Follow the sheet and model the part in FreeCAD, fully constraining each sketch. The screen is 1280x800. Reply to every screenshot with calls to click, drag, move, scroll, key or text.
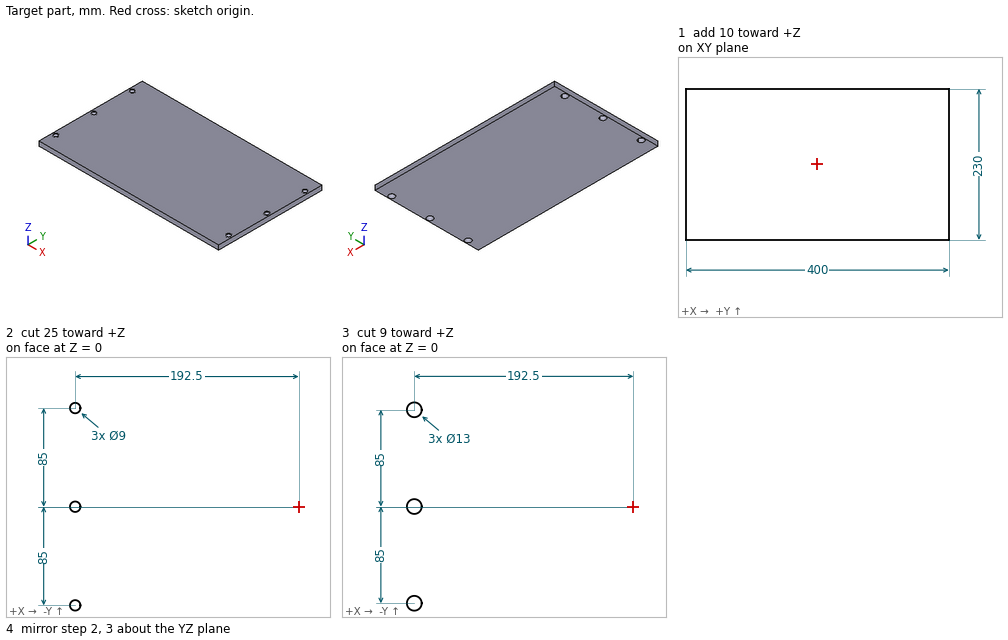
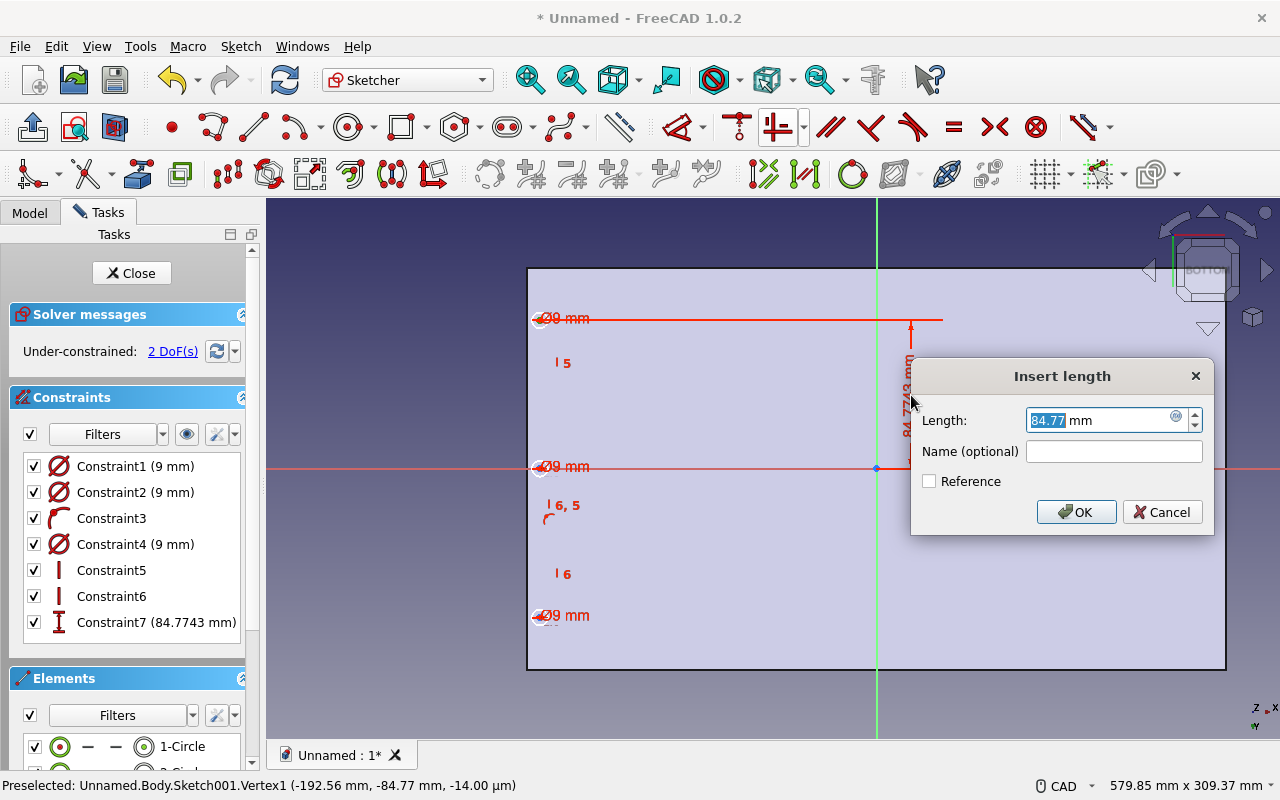
text(85)
key(Return)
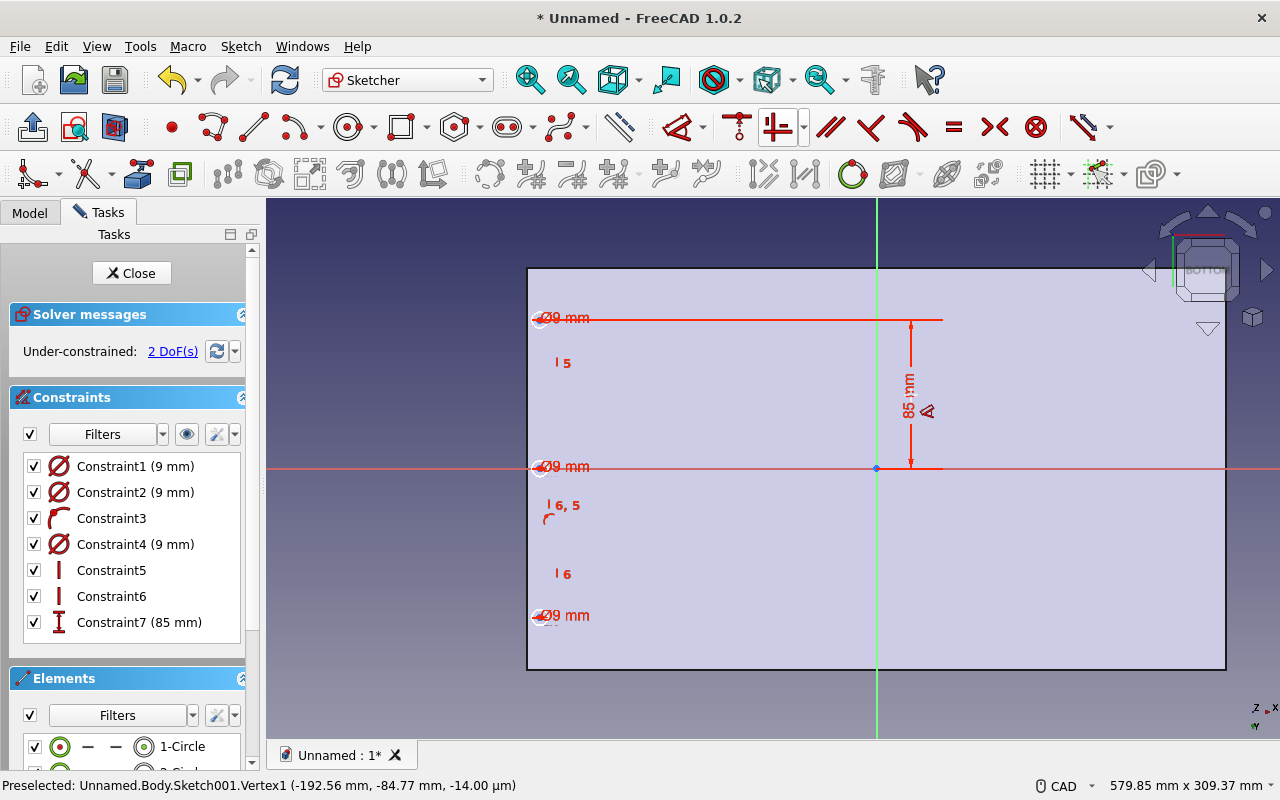
click(540, 618)
click(911, 543)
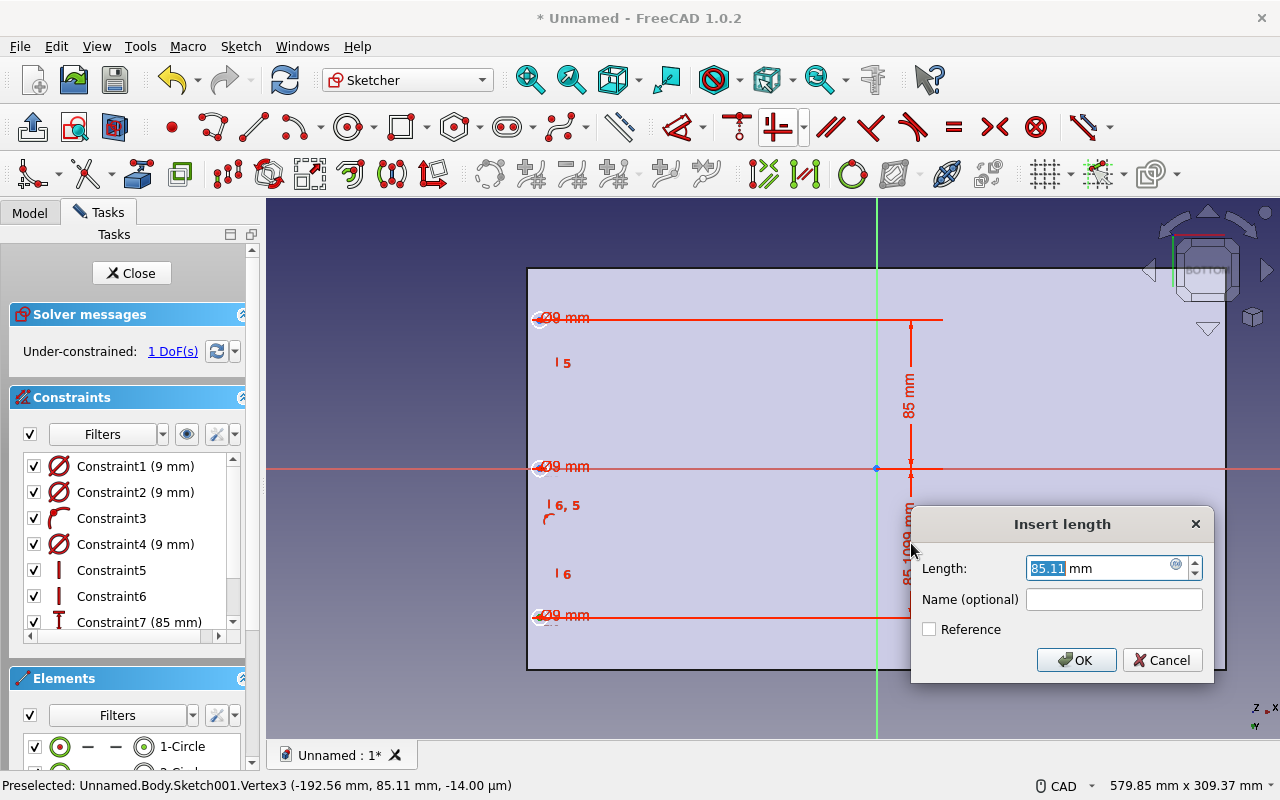
text(85)
key(Return)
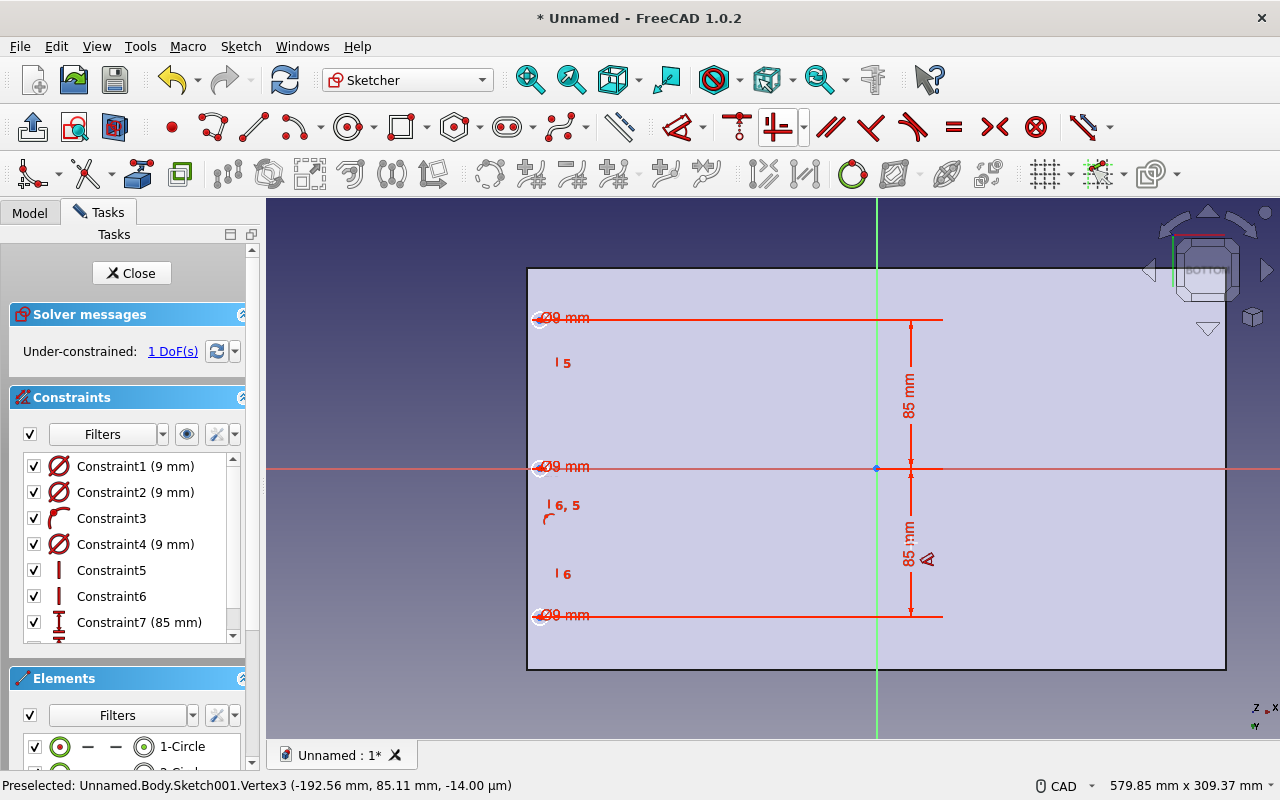
click(540, 320)
click(708, 286)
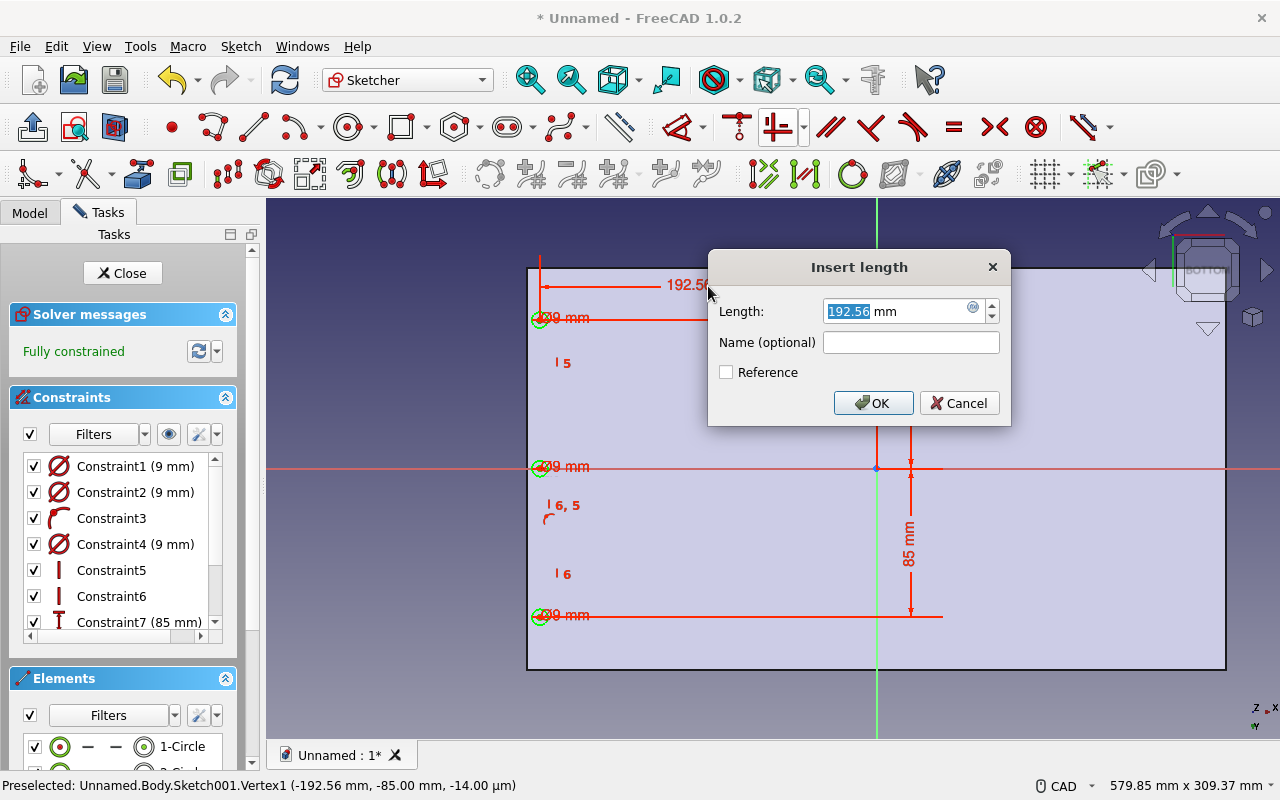
text(192.5)
key(Return)
key(Escape)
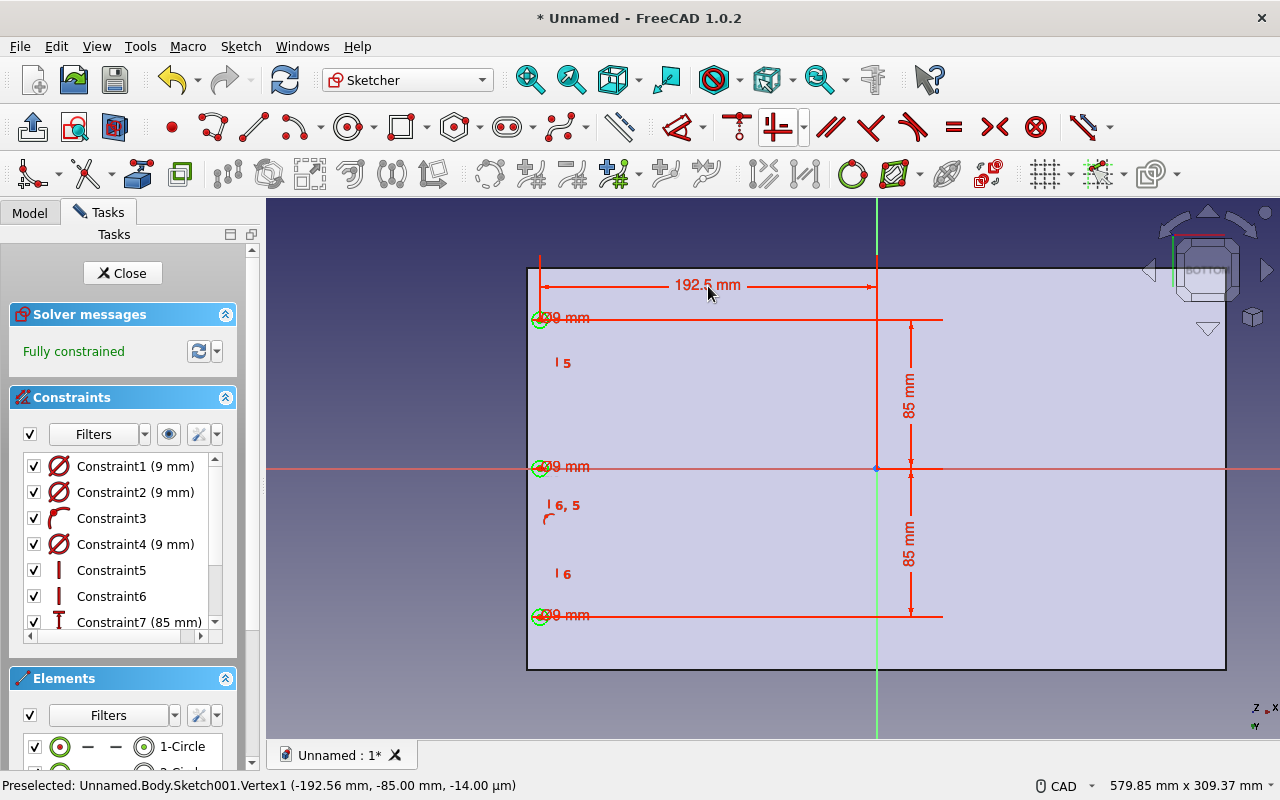
click(123, 273)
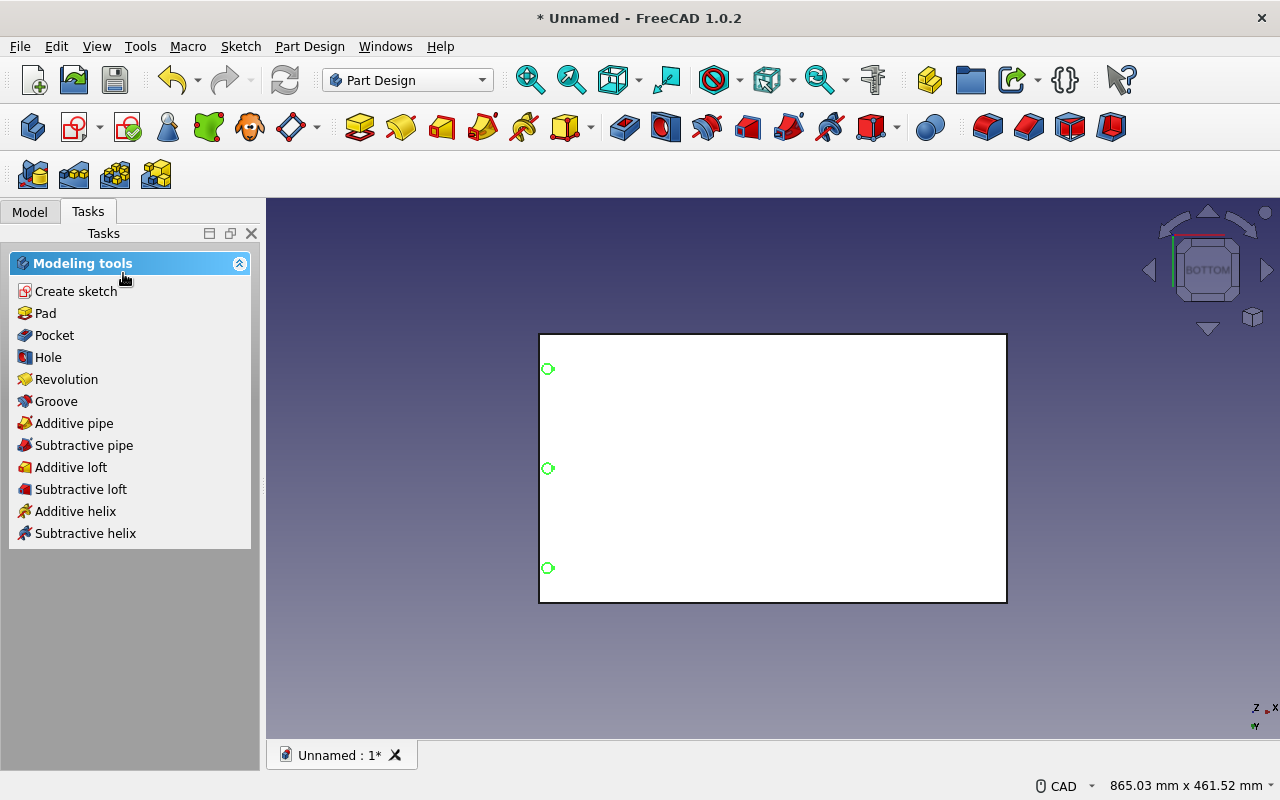
click(625, 128)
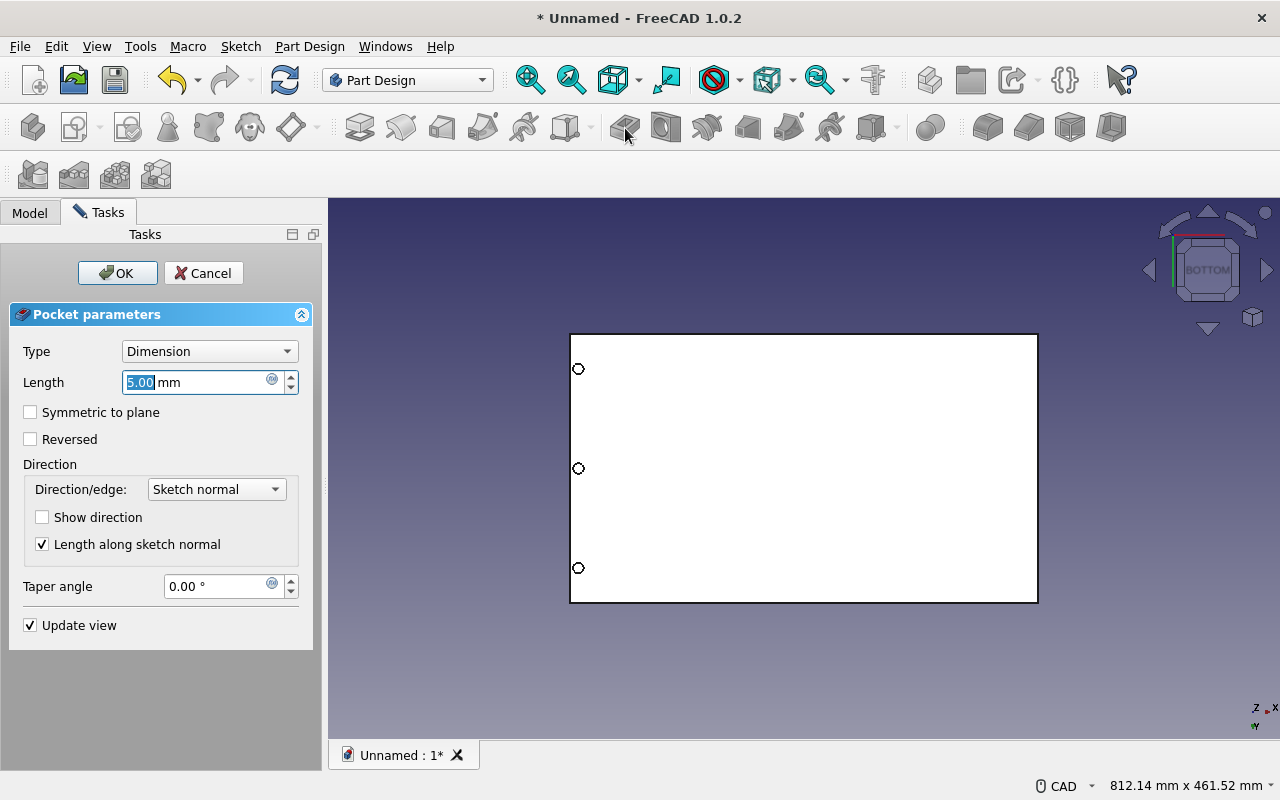
text(25)
key(Tab)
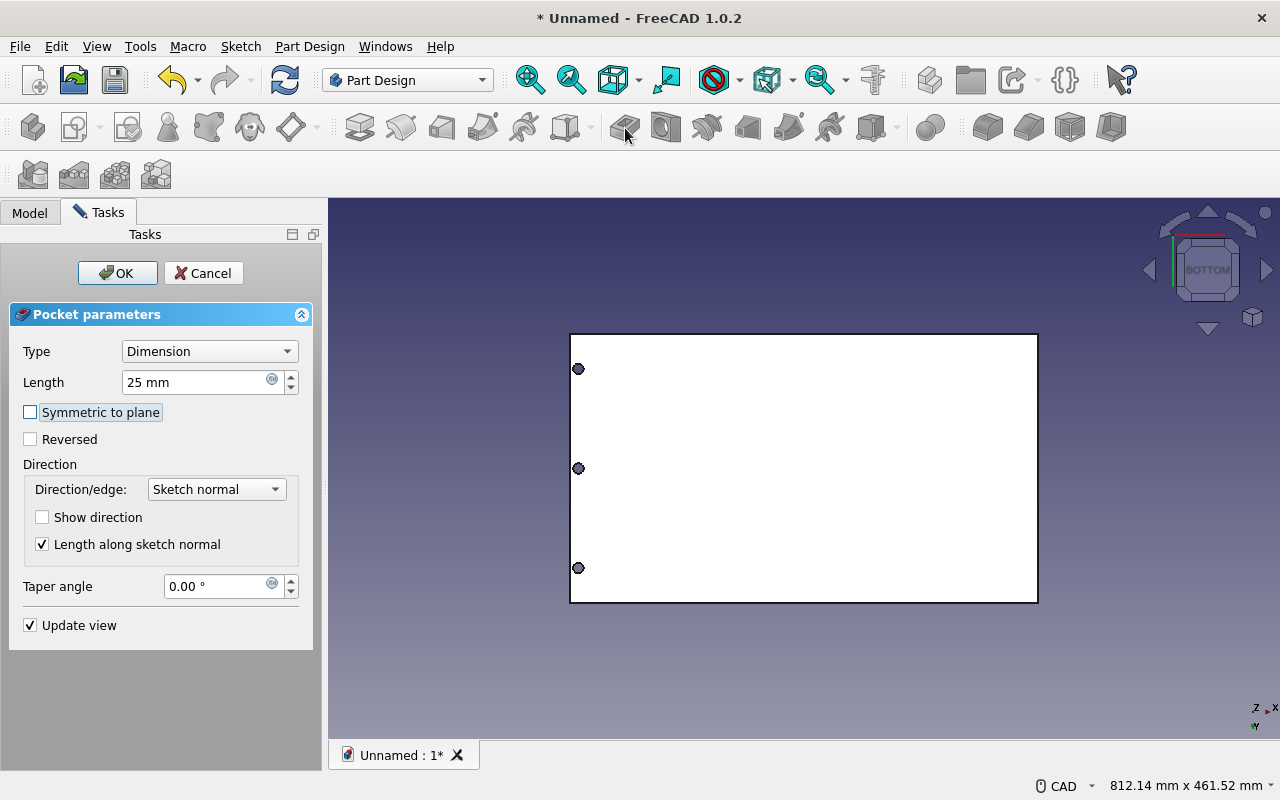
click(118, 273)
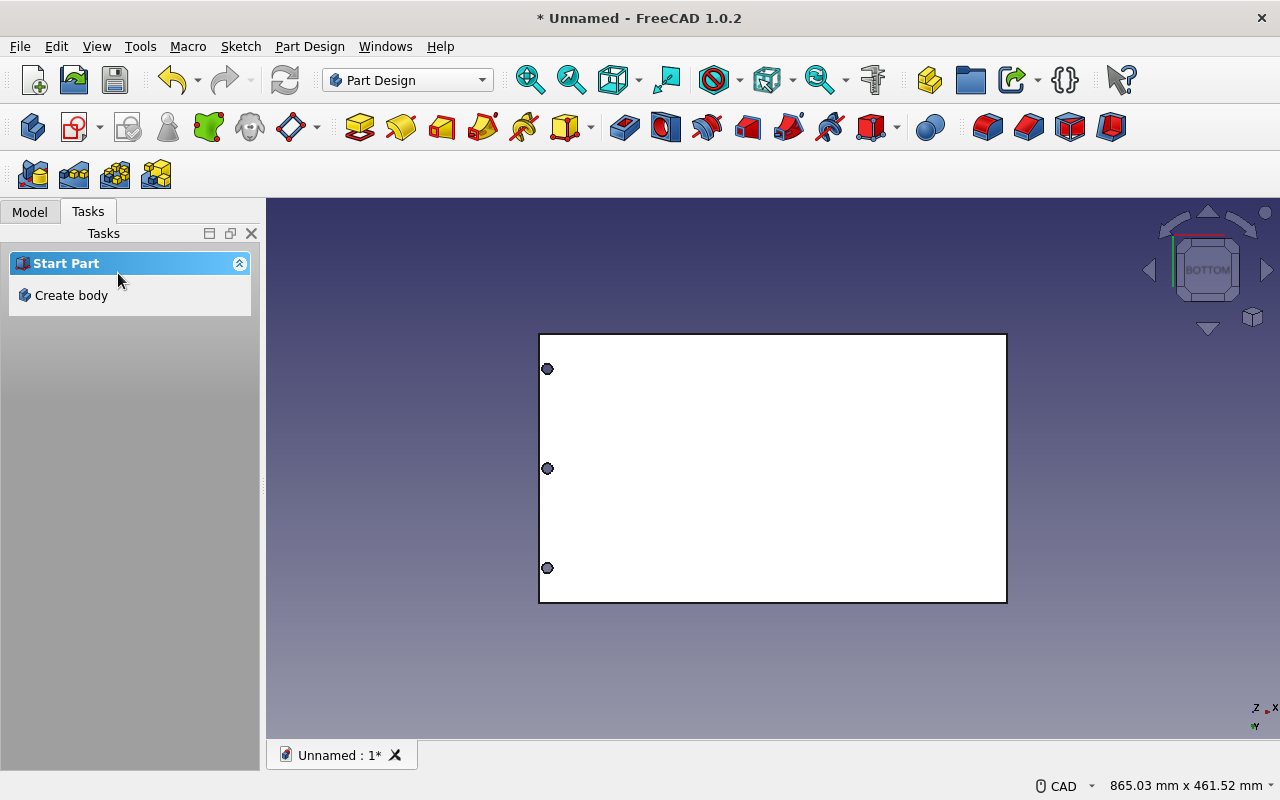
click(840, 468)